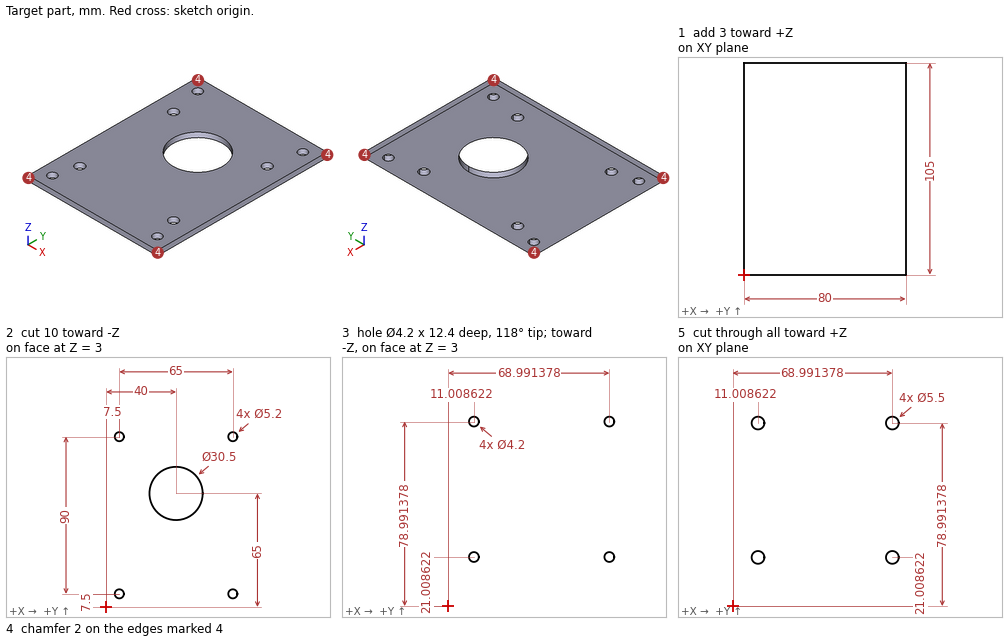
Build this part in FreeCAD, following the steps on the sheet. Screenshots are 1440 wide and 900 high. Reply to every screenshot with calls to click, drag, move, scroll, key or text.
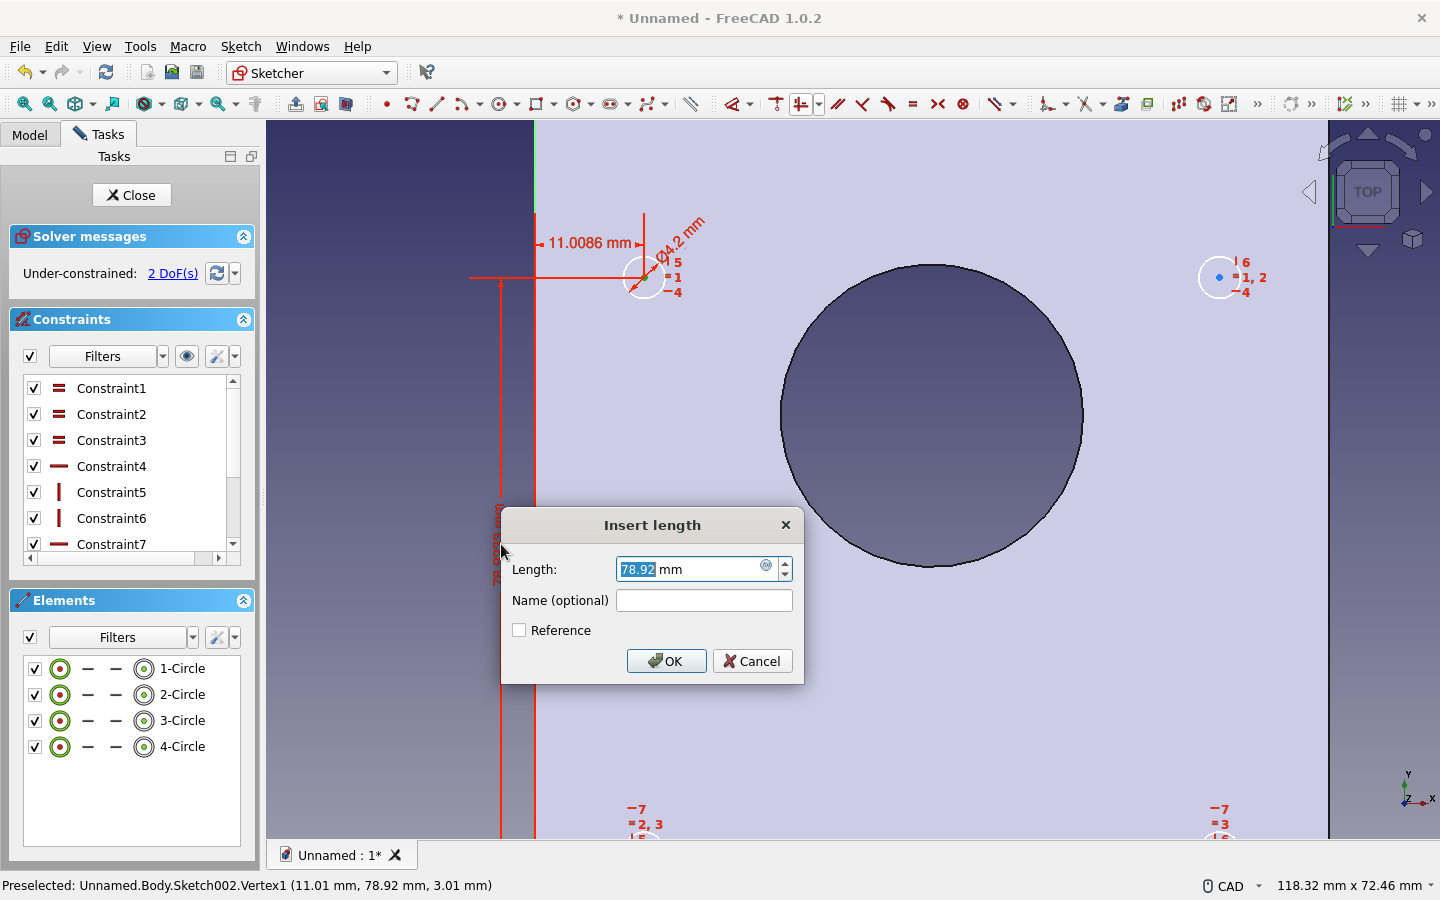
text(78.991378)
key(Return)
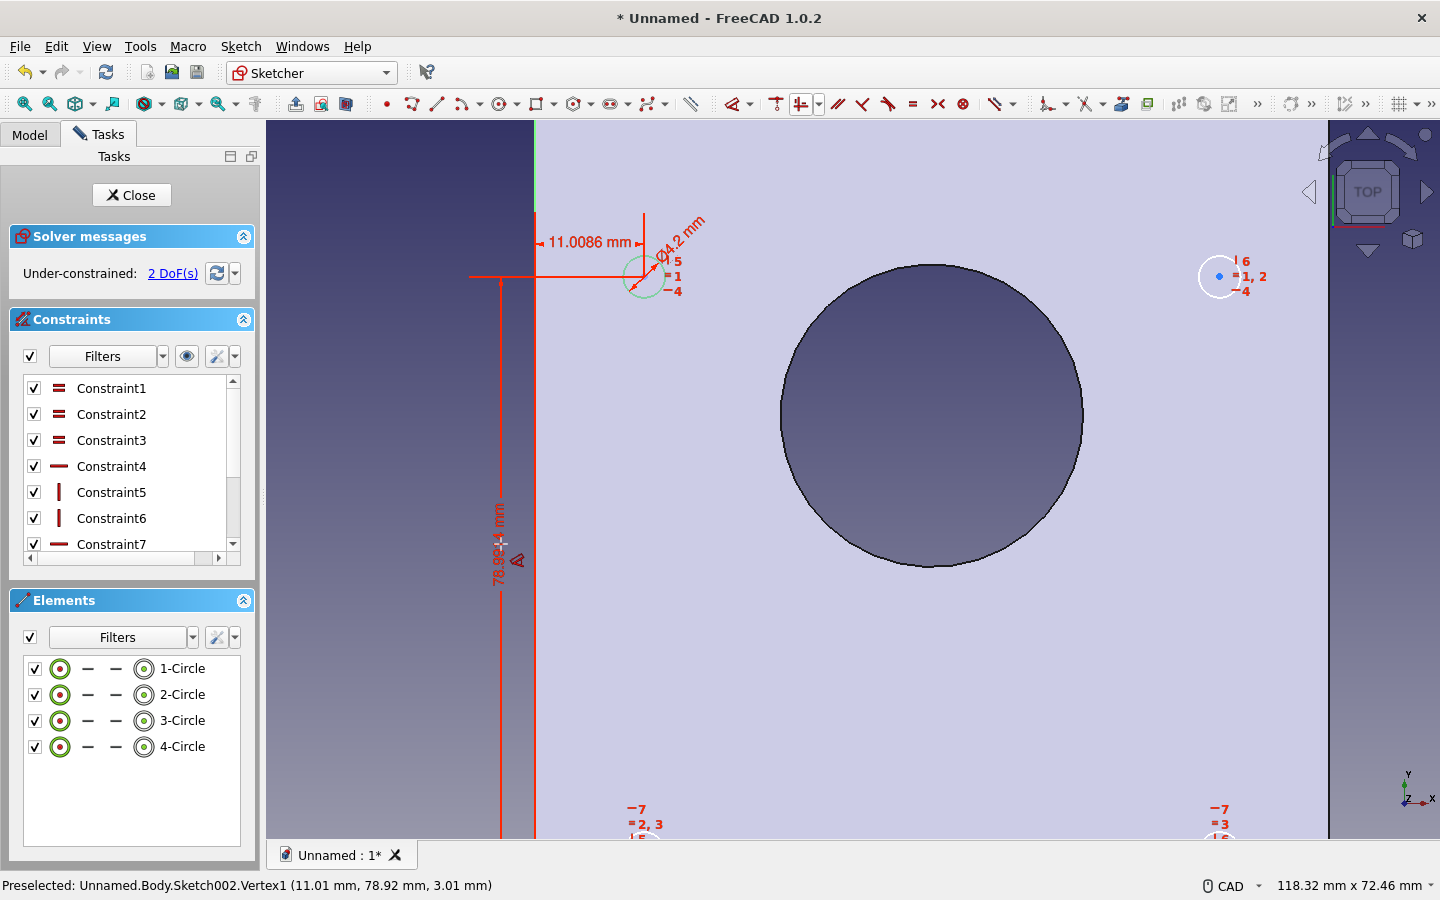
click(1220, 277)
click(877, 243)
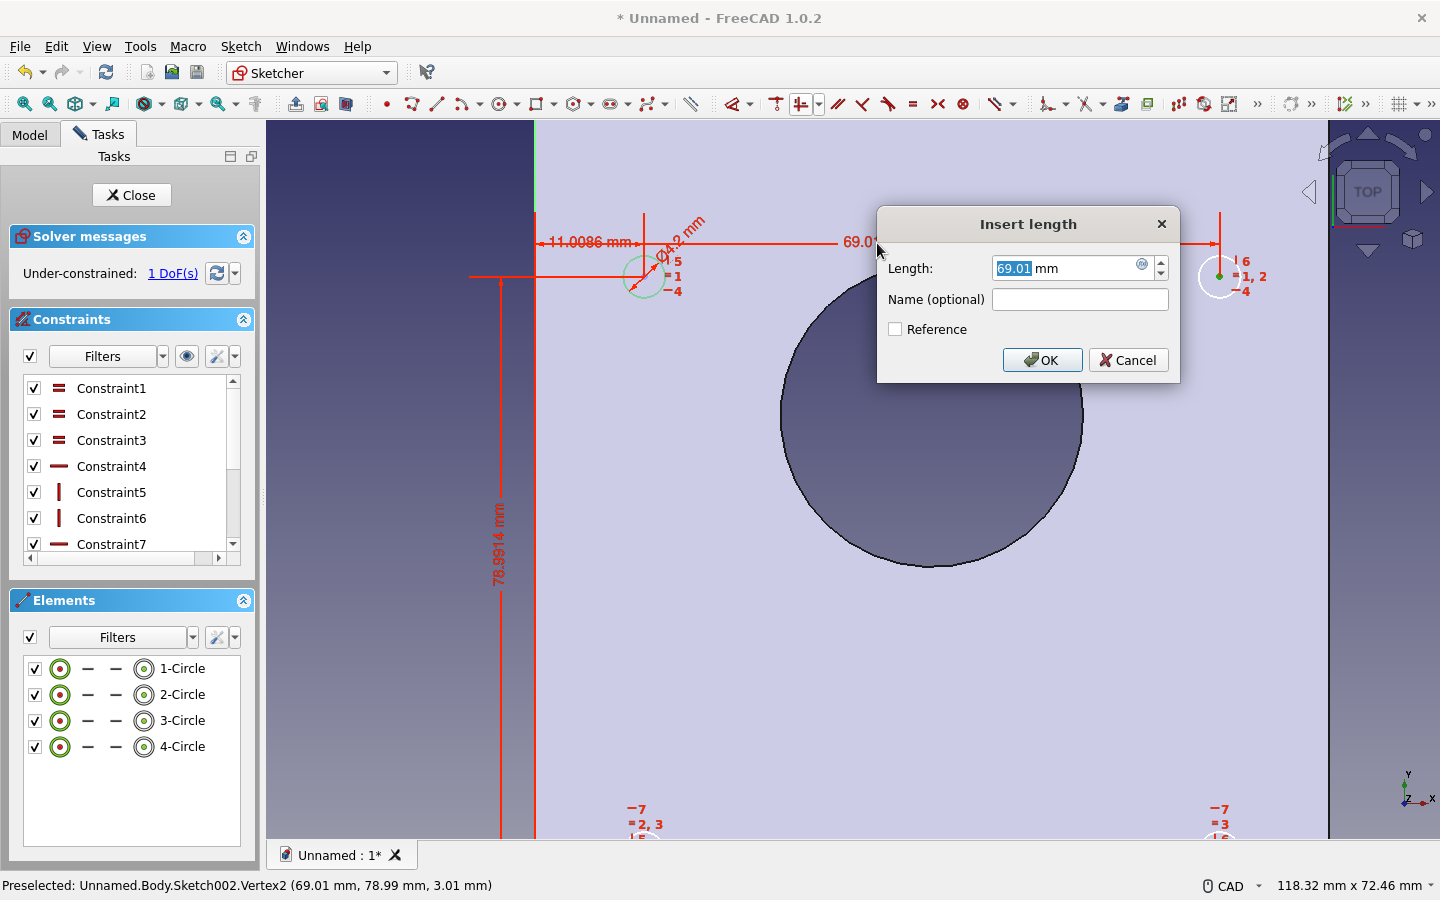
text(68.991378)
key(Return)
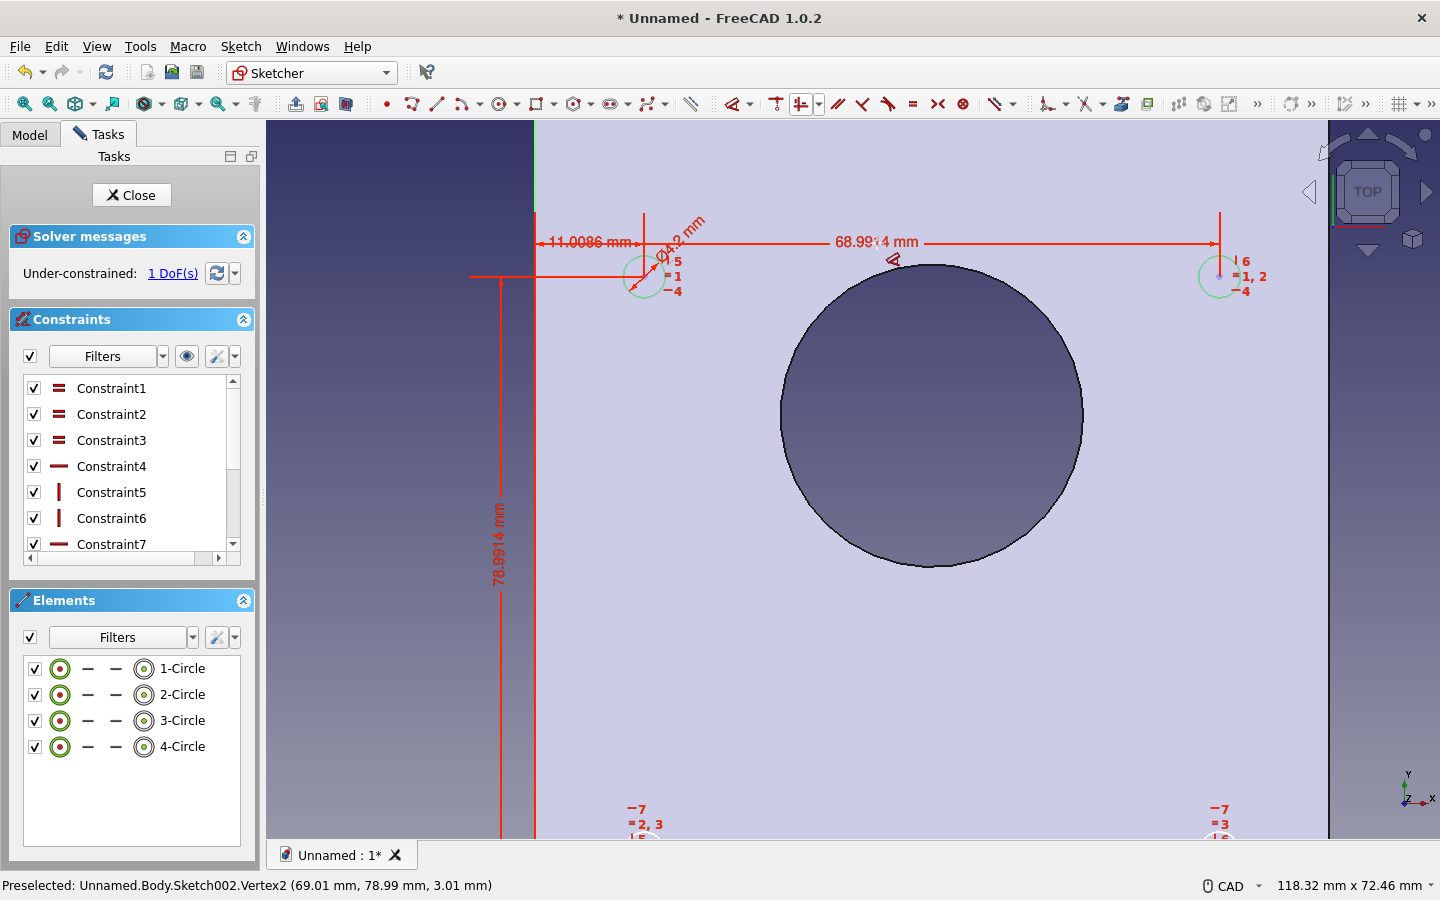
scroll(659, 262, down, 3)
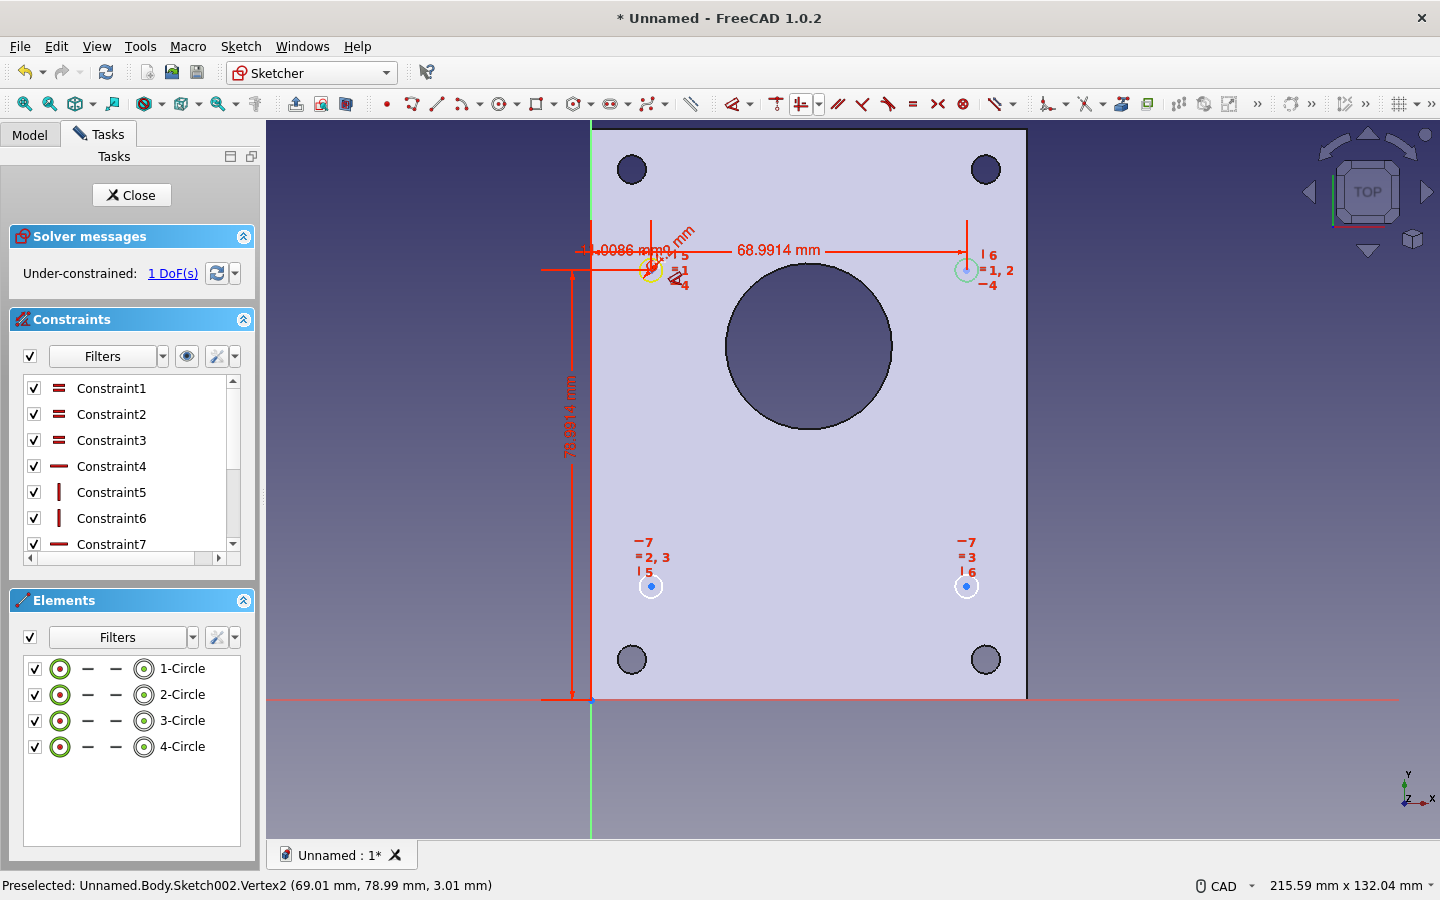
click(651, 586)
click(557, 643)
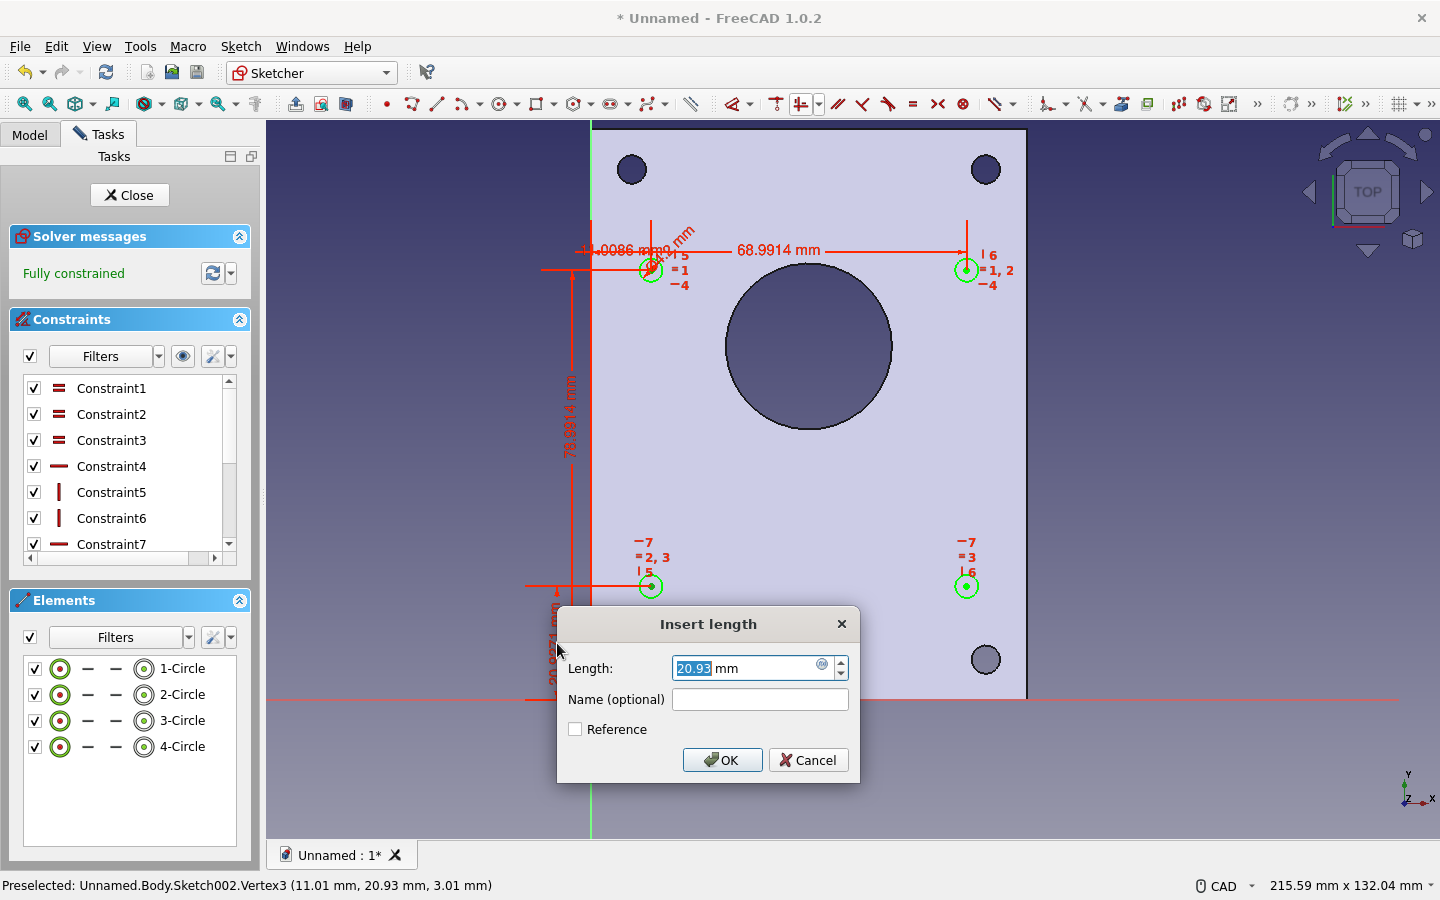
text(21.008622)
key(Return)
key(Escape)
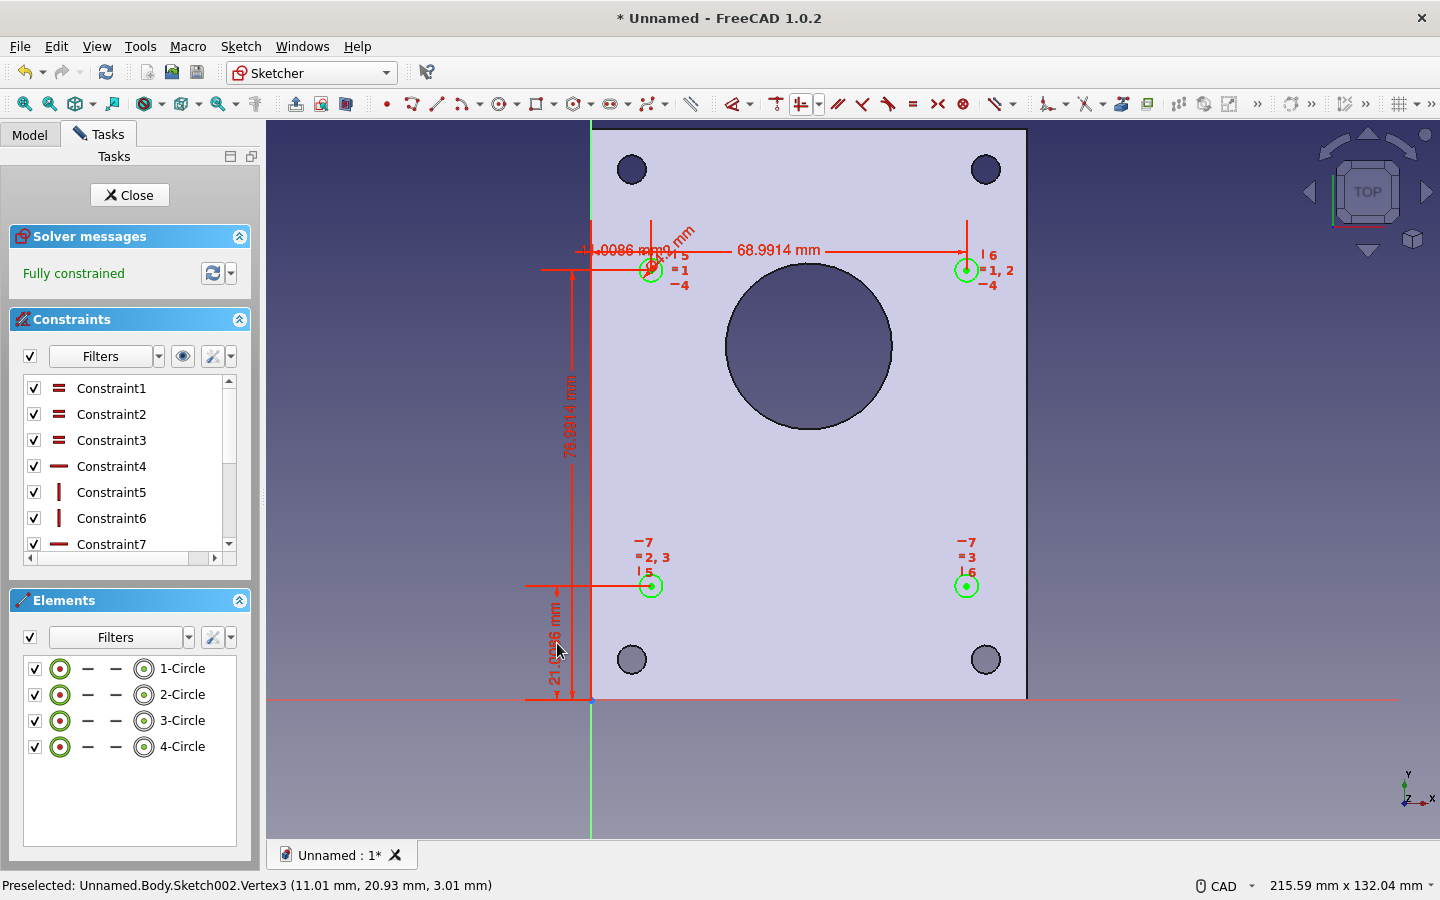
click(130, 195)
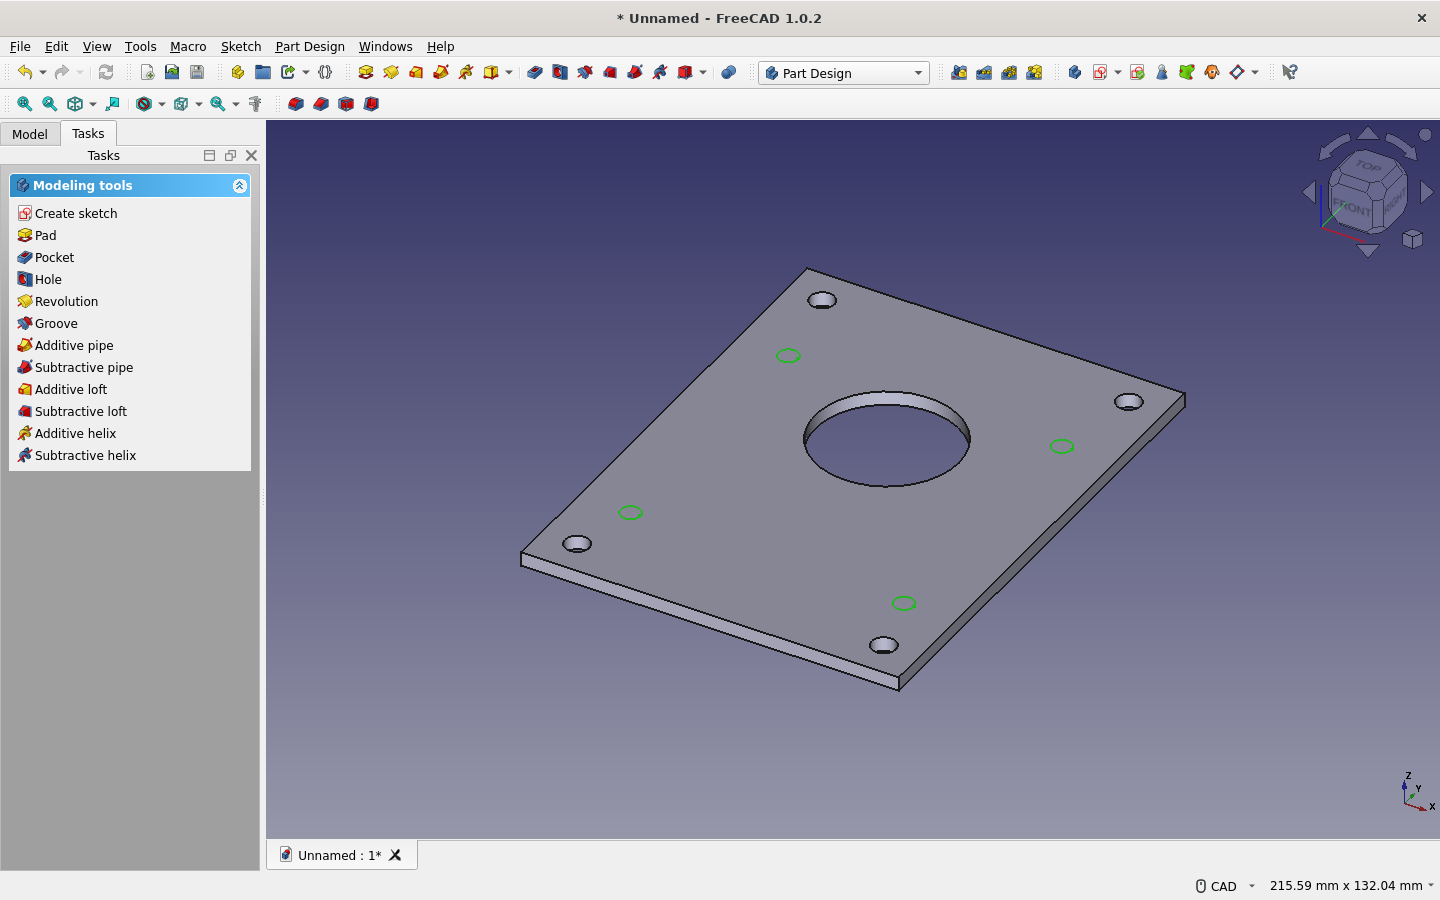
click(560, 72)